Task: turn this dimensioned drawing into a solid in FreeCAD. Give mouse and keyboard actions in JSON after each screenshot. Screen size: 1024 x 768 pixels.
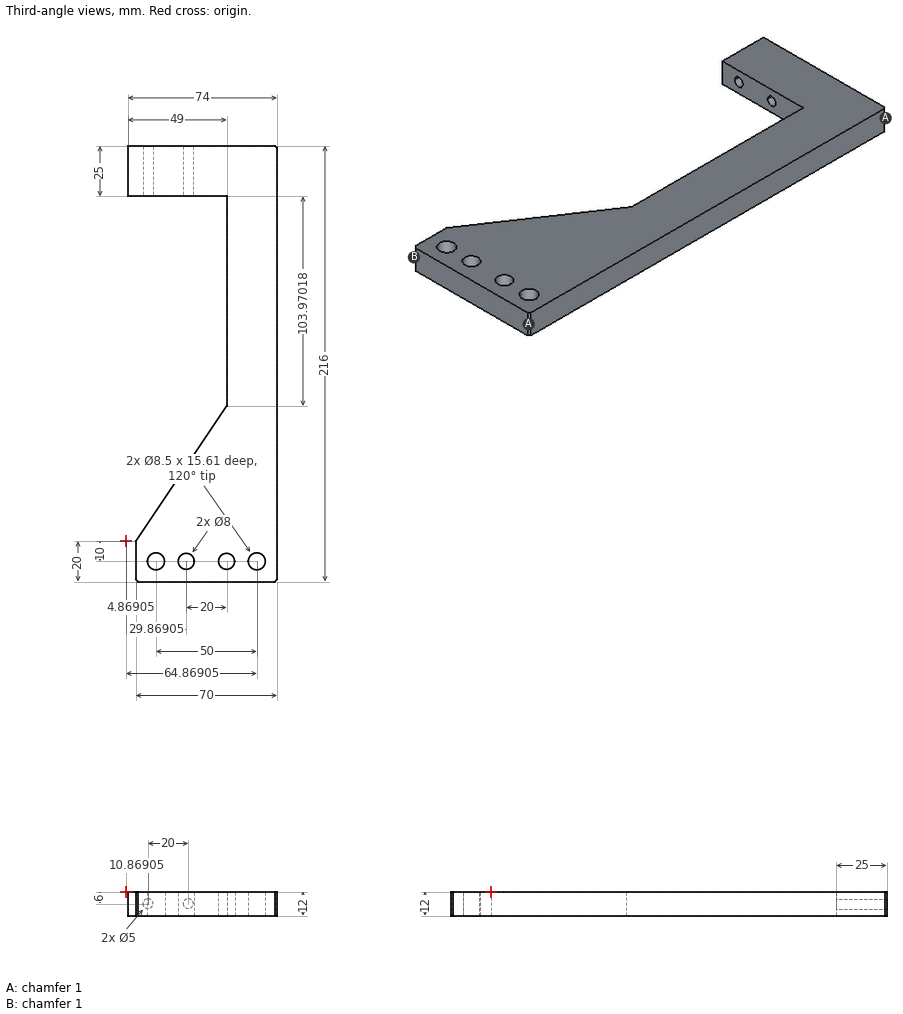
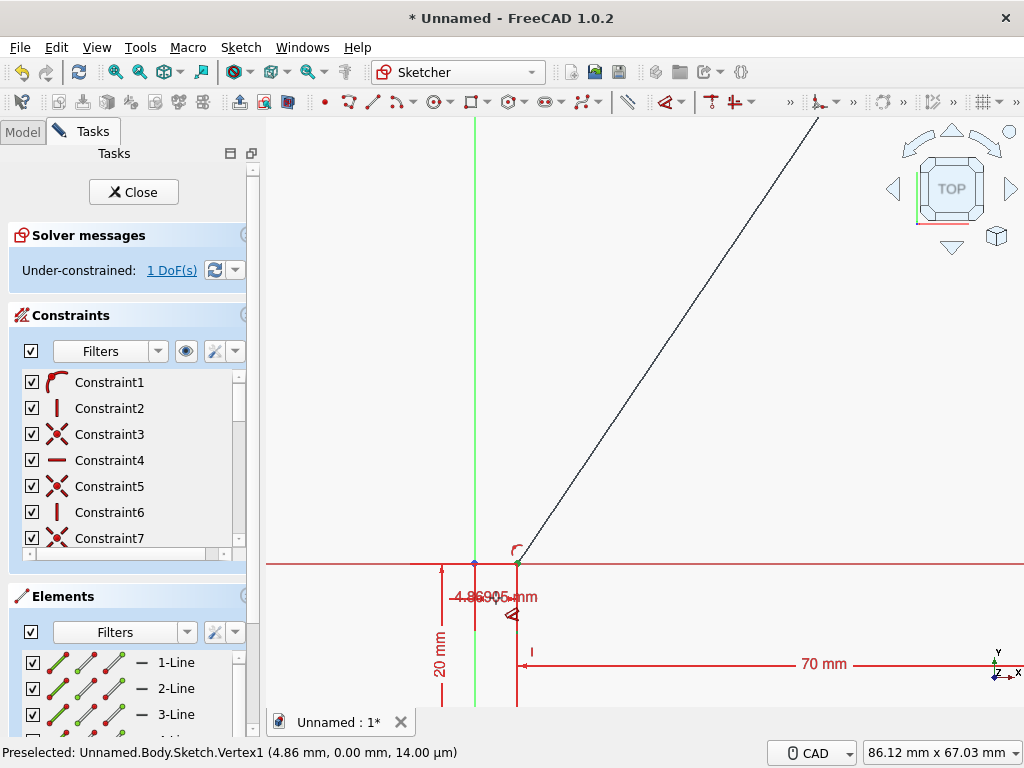
{"action": "scroll", "coordinate": [519, 569], "scroll_direction": "down", "scroll_amount": 8}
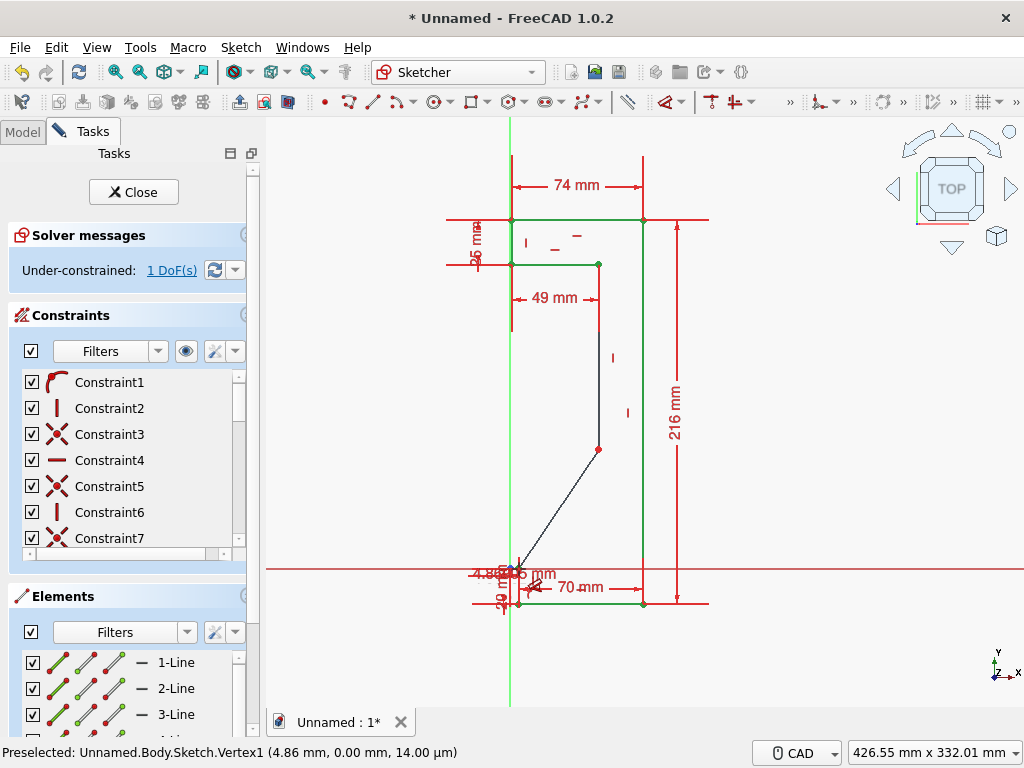
{"action": "left_click", "coordinate": [599, 320]}
{"action": "left_click", "coordinate": [565, 357]}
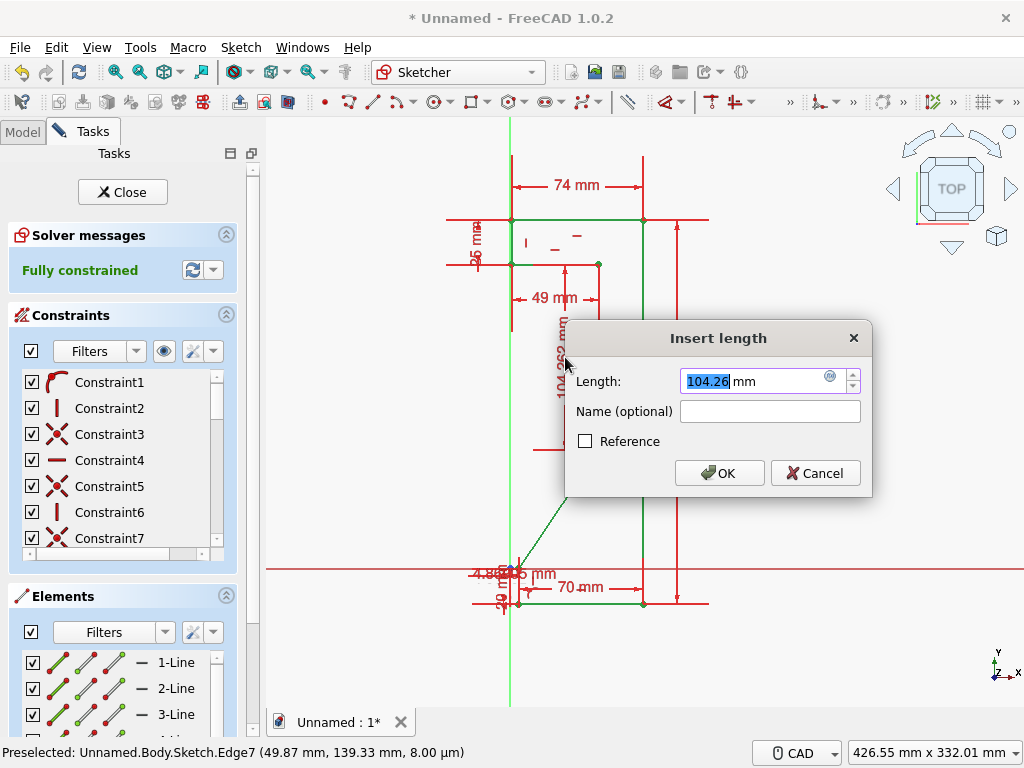
{"action": "type", "text": "103.97018"}
{"action": "key", "text": "Return"}
{"action": "key", "text": "Escape"}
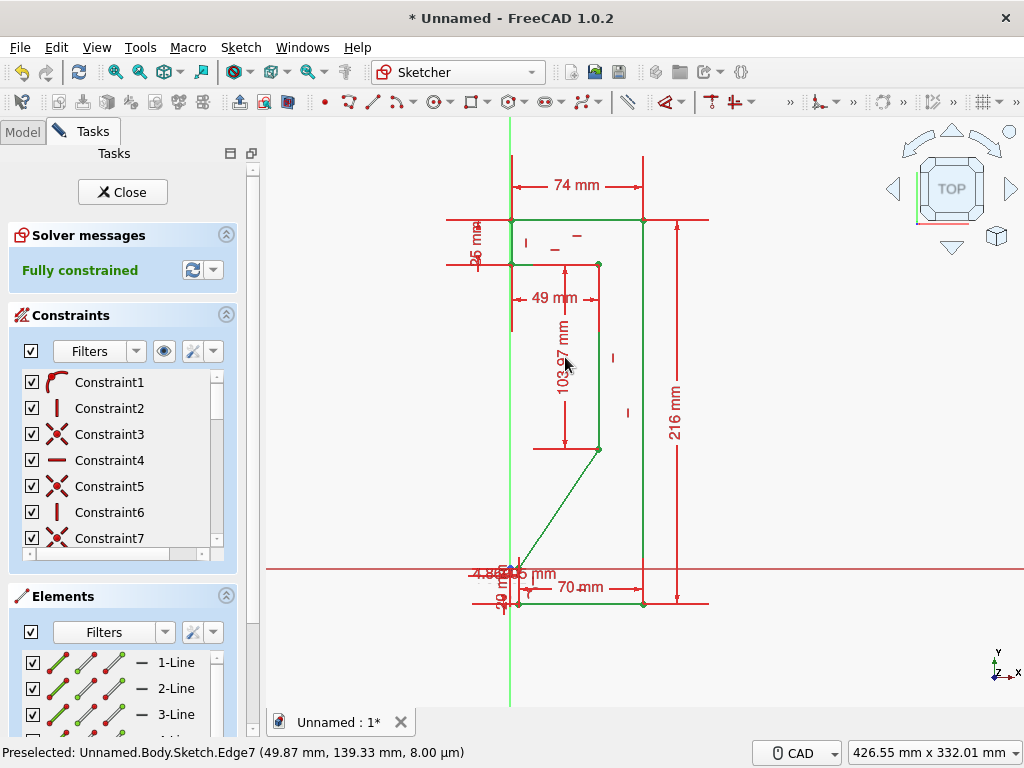
{"action": "left_click", "coordinate": [123, 192]}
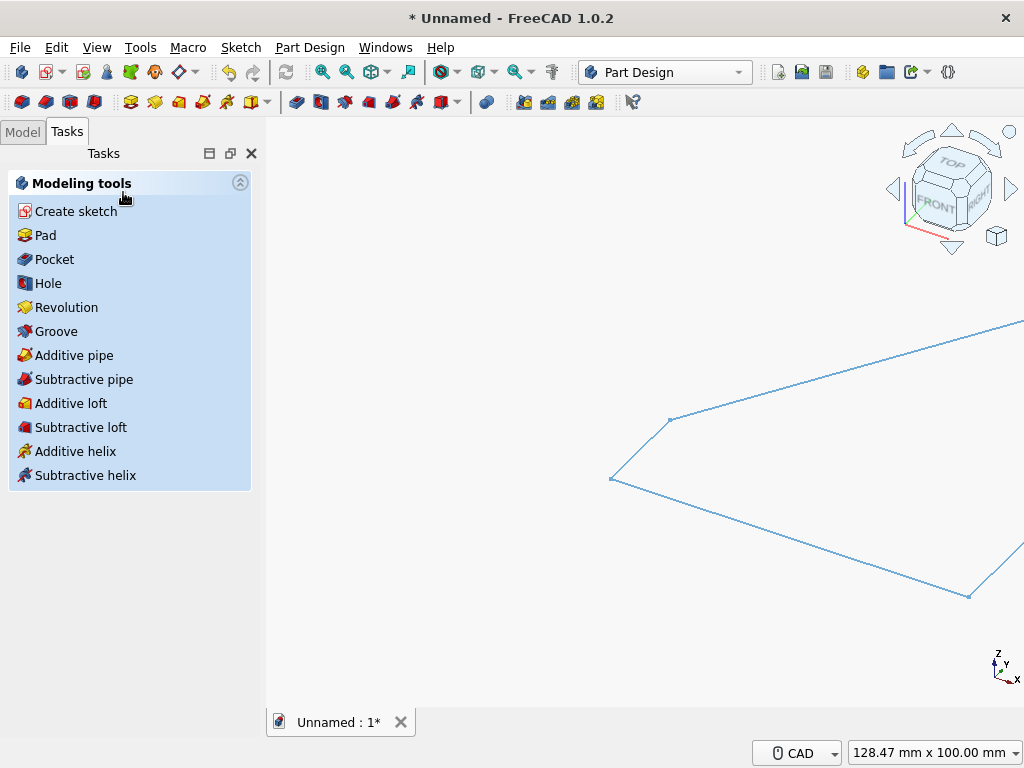
{"action": "left_click", "coordinate": [132, 102]}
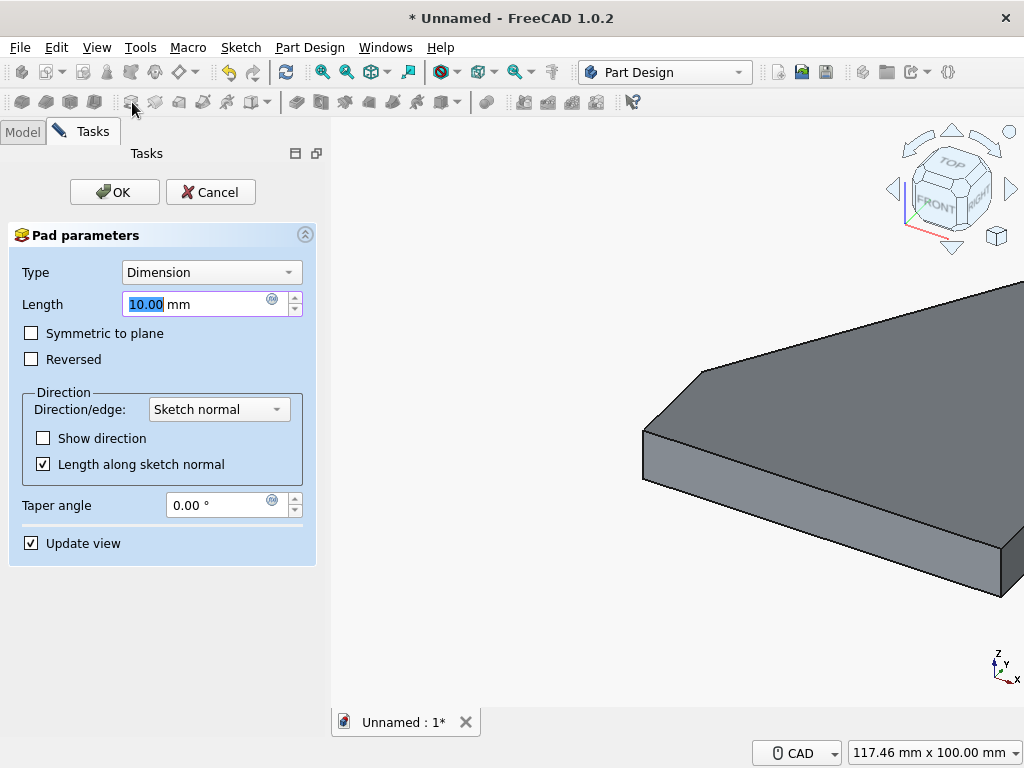
{"action": "type", "text": "12"}
{"action": "key", "text": "Tab"}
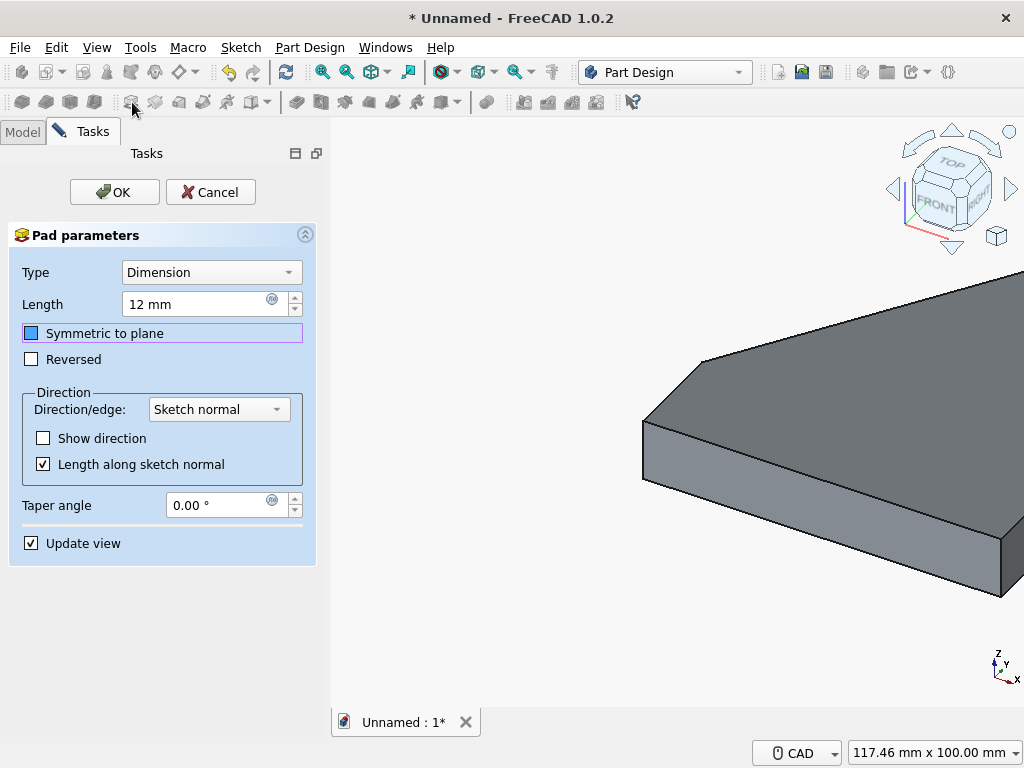
{"action": "left_click", "coordinate": [30, 359]}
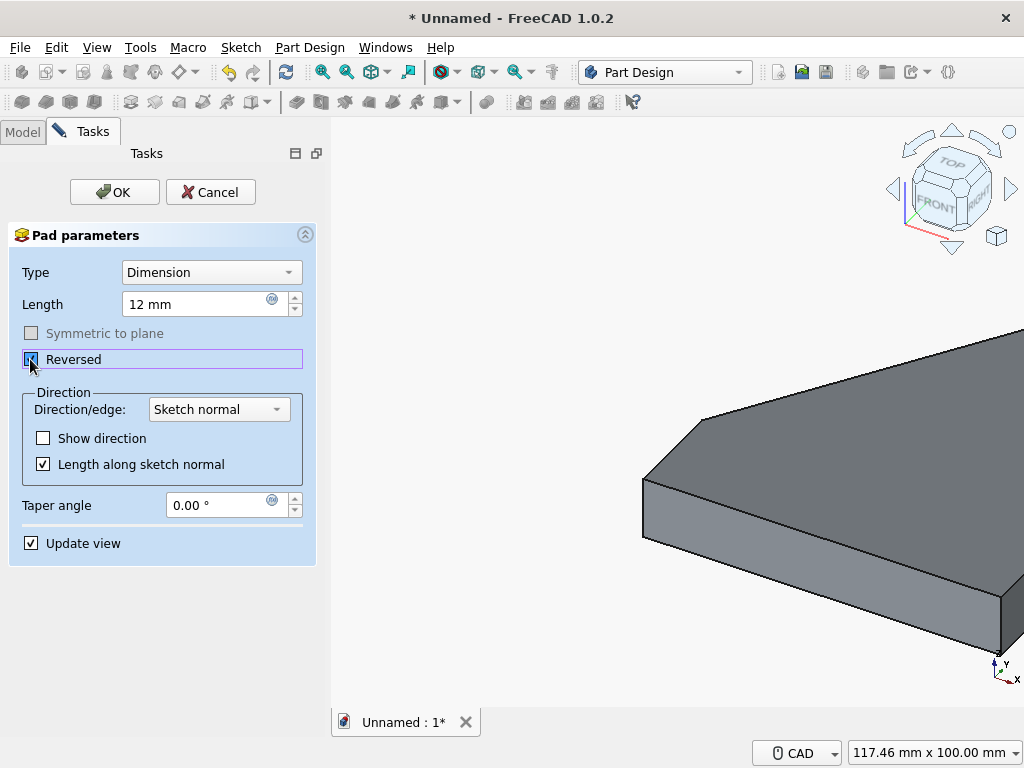
{"action": "left_click", "coordinate": [115, 192]}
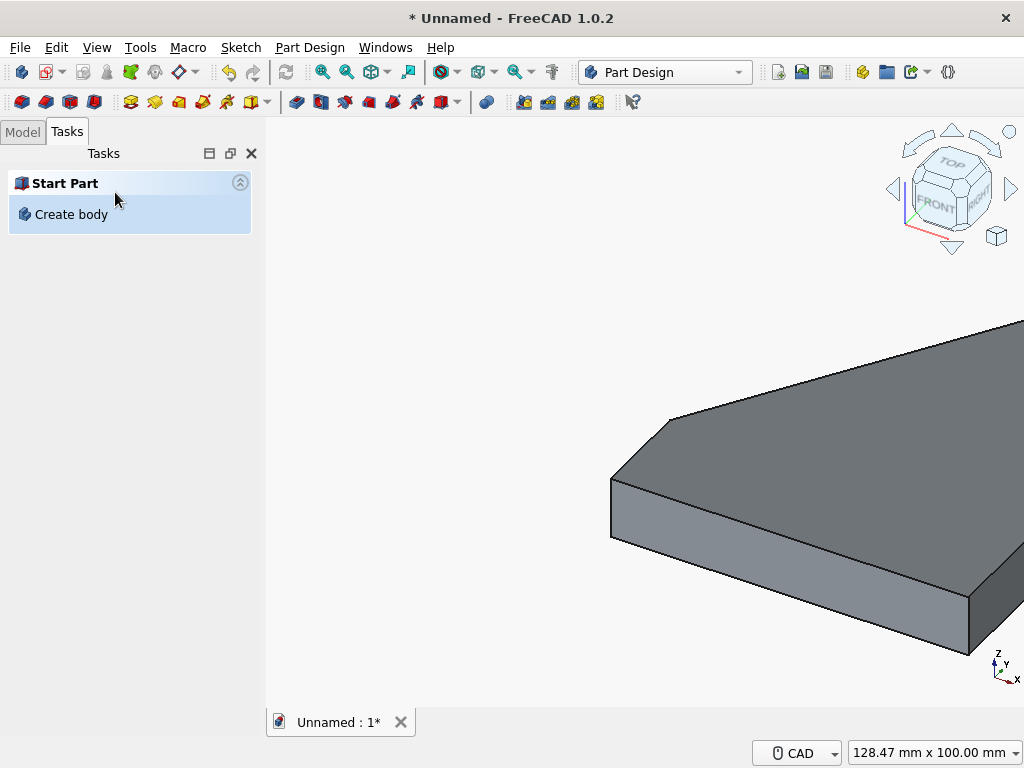
{"action": "key", "text": "v f"}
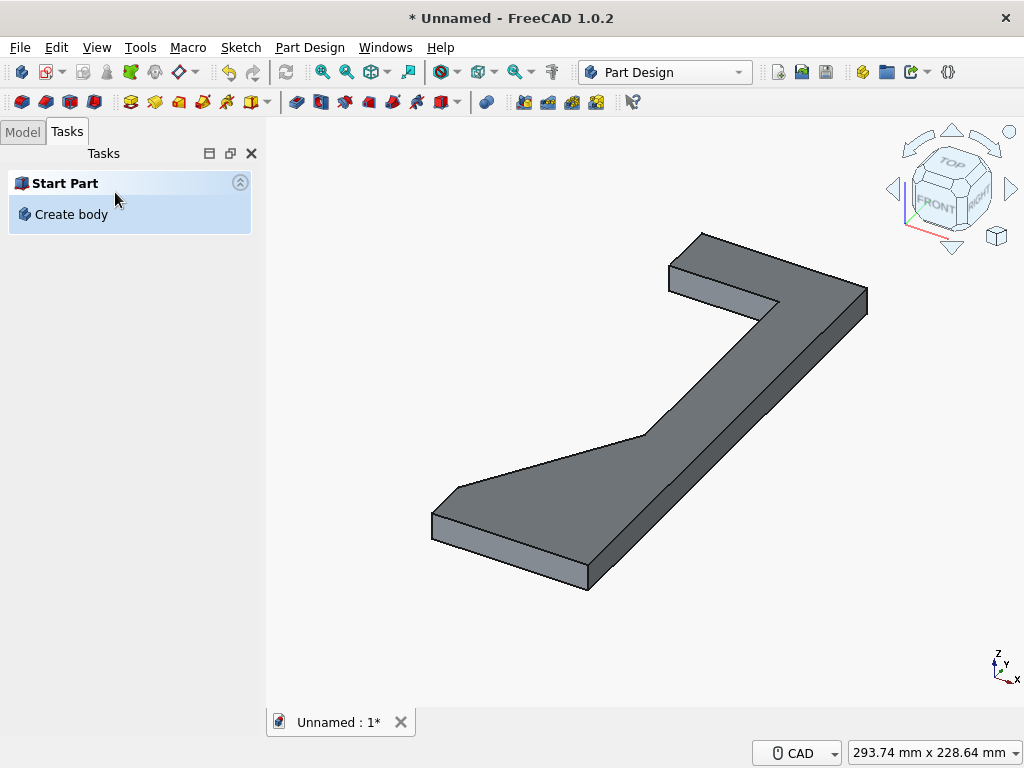
{"action": "left_click", "coordinate": [589, 485]}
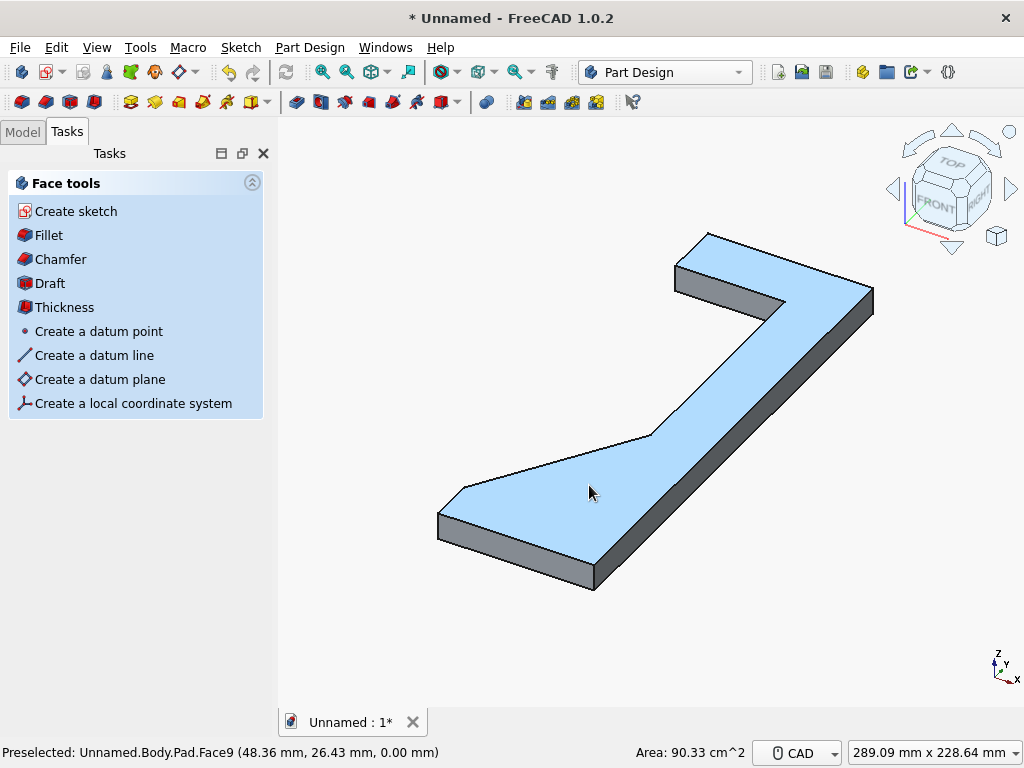
{"action": "left_click", "coordinate": [46, 72]}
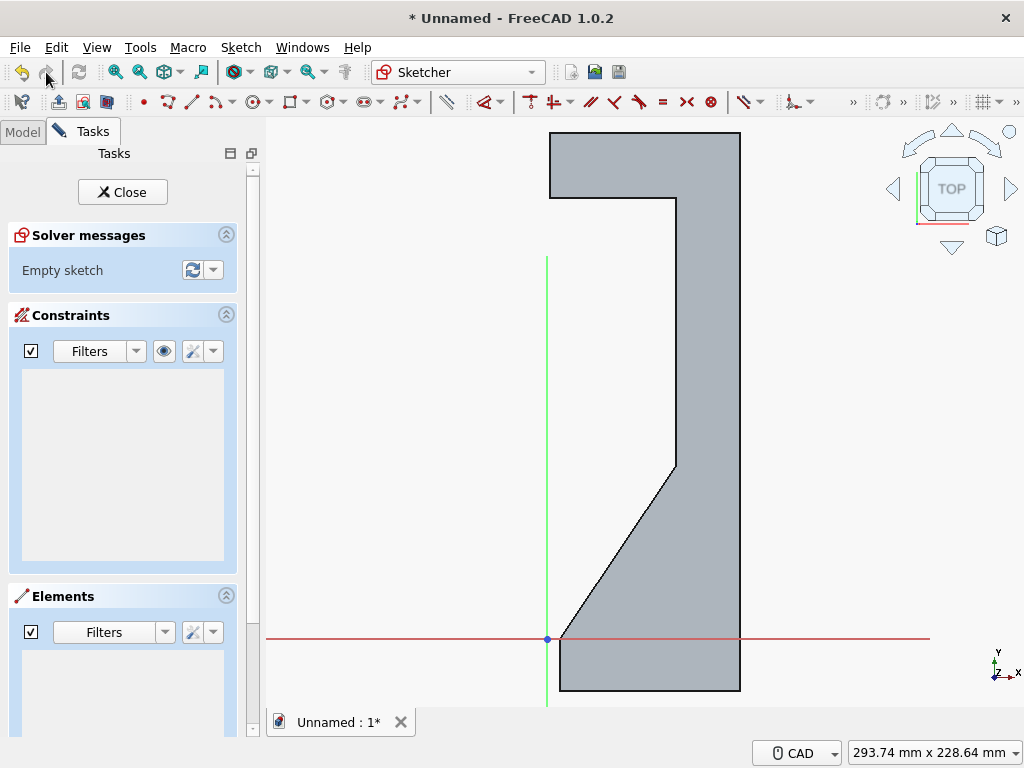
{"action": "scroll", "coordinate": [576, 412], "scroll_direction": "down", "scroll_amount": 5}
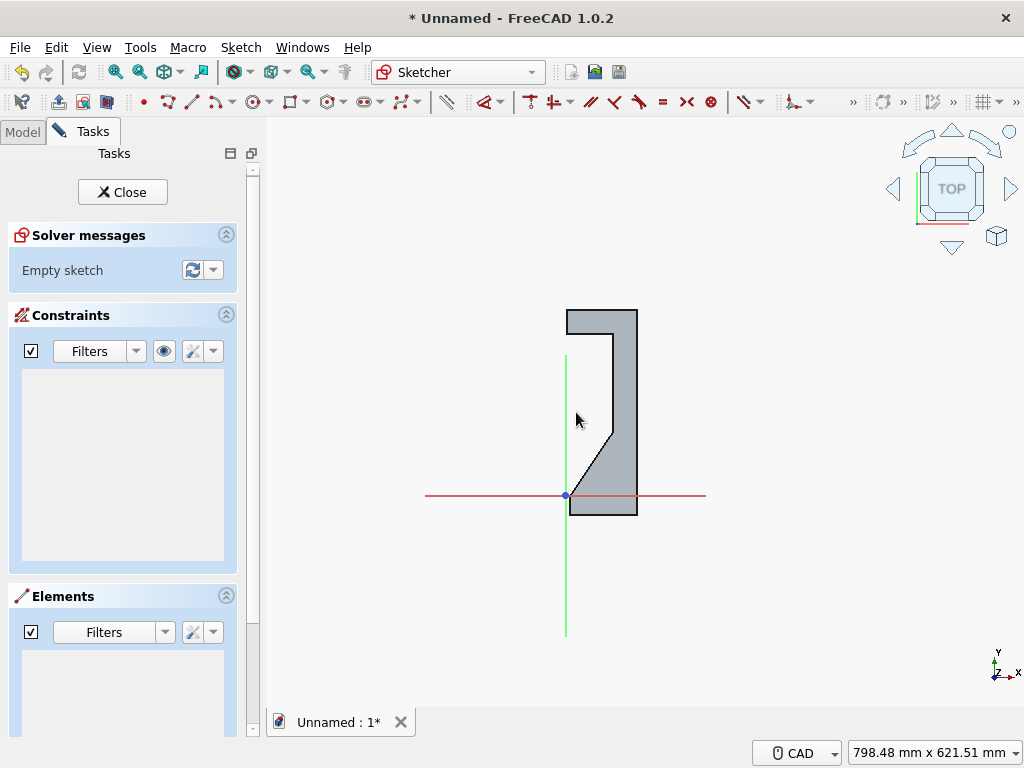
{"action": "scroll", "coordinate": [603, 521], "scroll_direction": "up", "scroll_amount": 9}